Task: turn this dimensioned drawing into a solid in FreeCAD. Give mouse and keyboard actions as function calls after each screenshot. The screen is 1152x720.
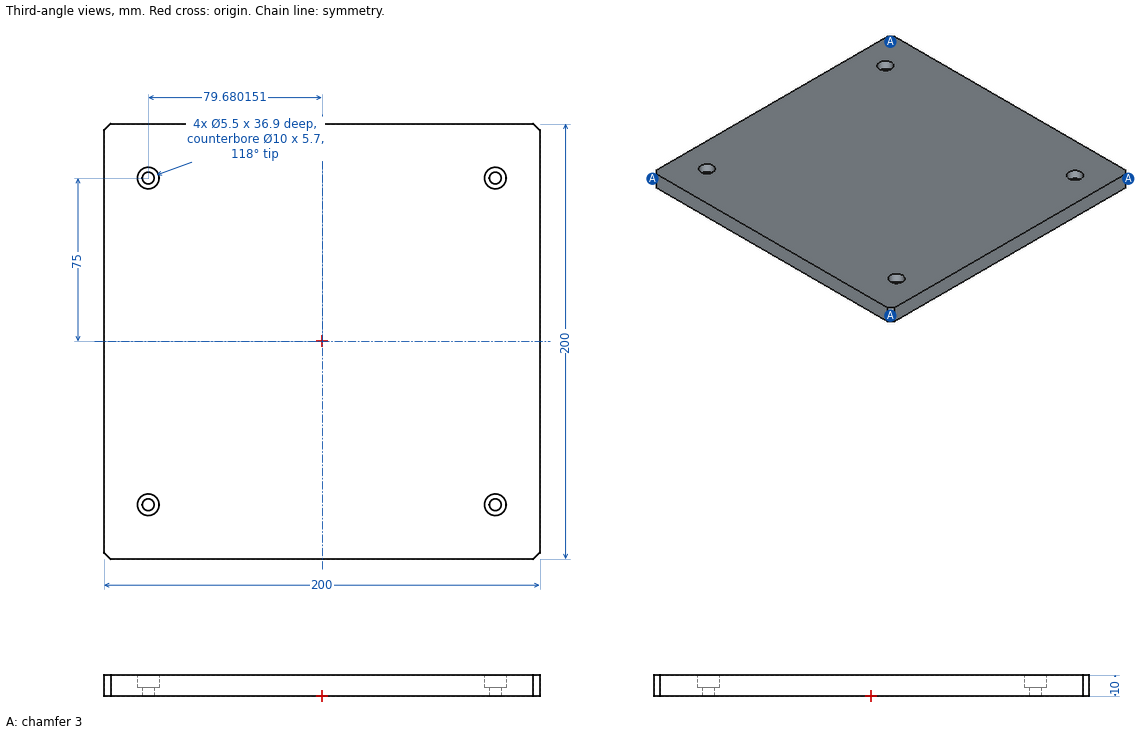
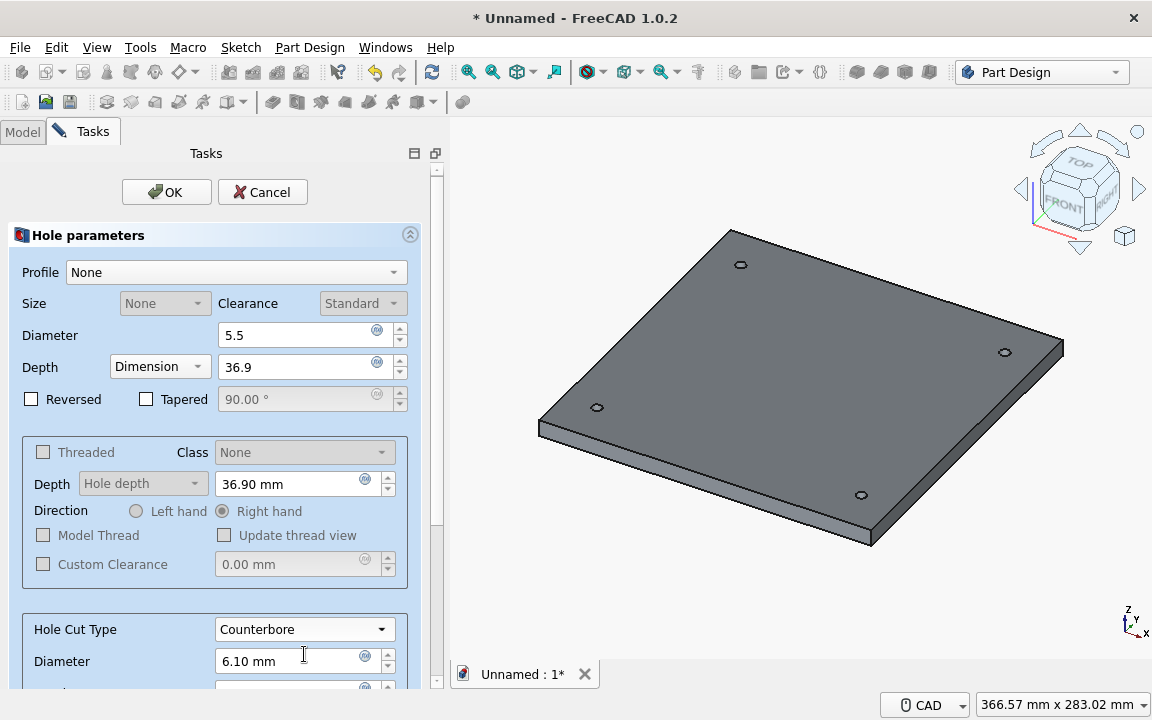
triple_click(298, 661)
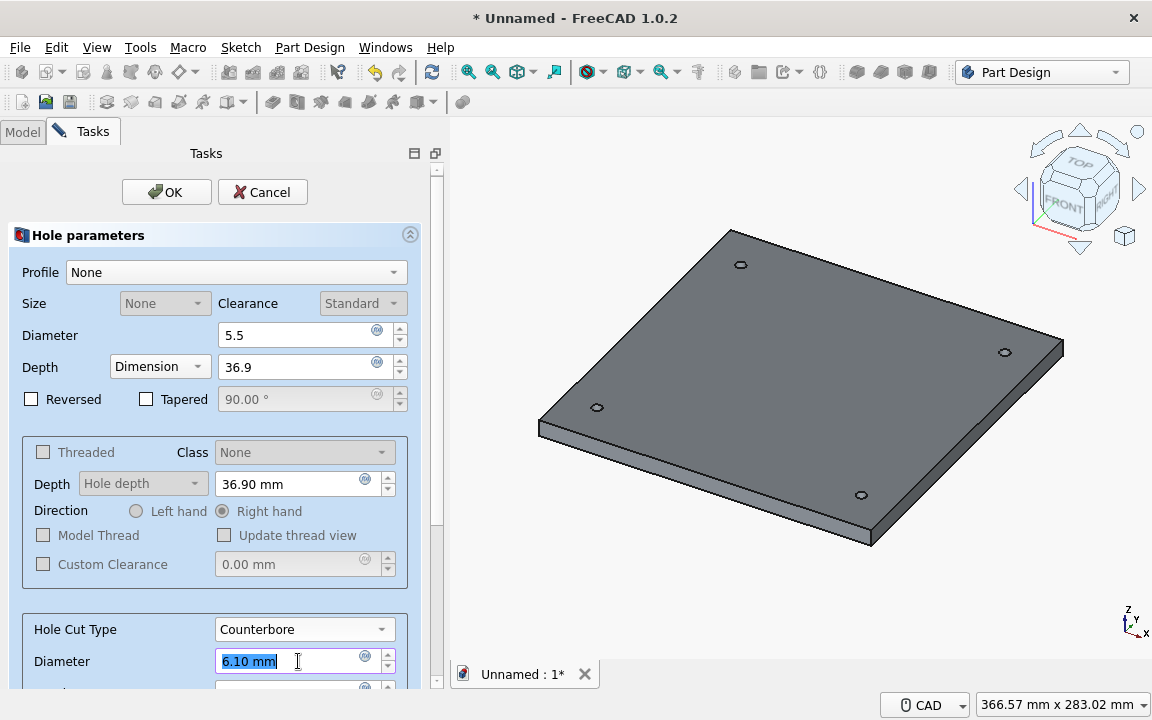
text(10)
key(Tab)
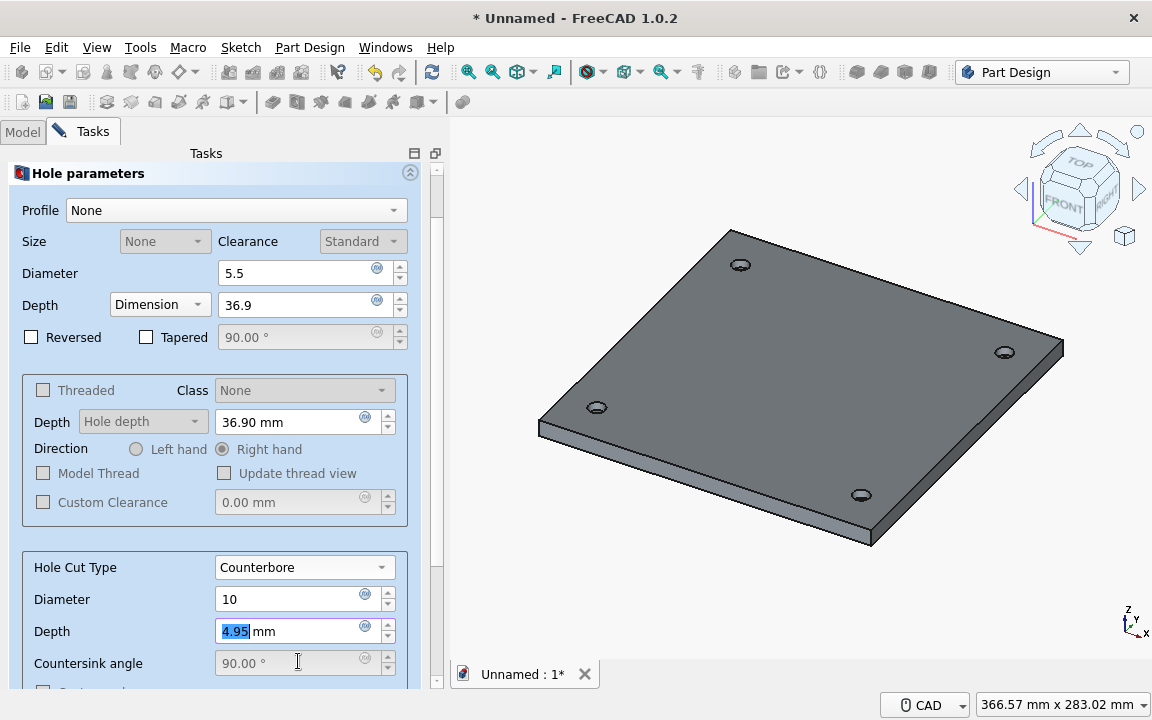
text(5.7)
key(Tab)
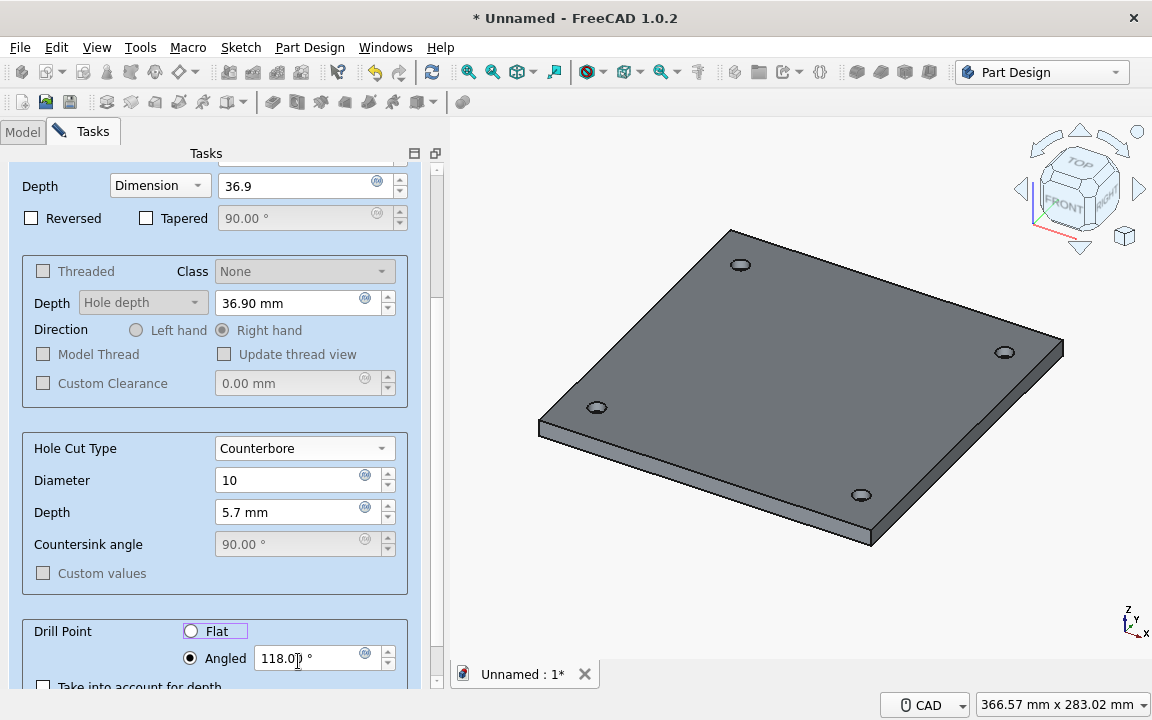
scroll(437, 426, up, 4)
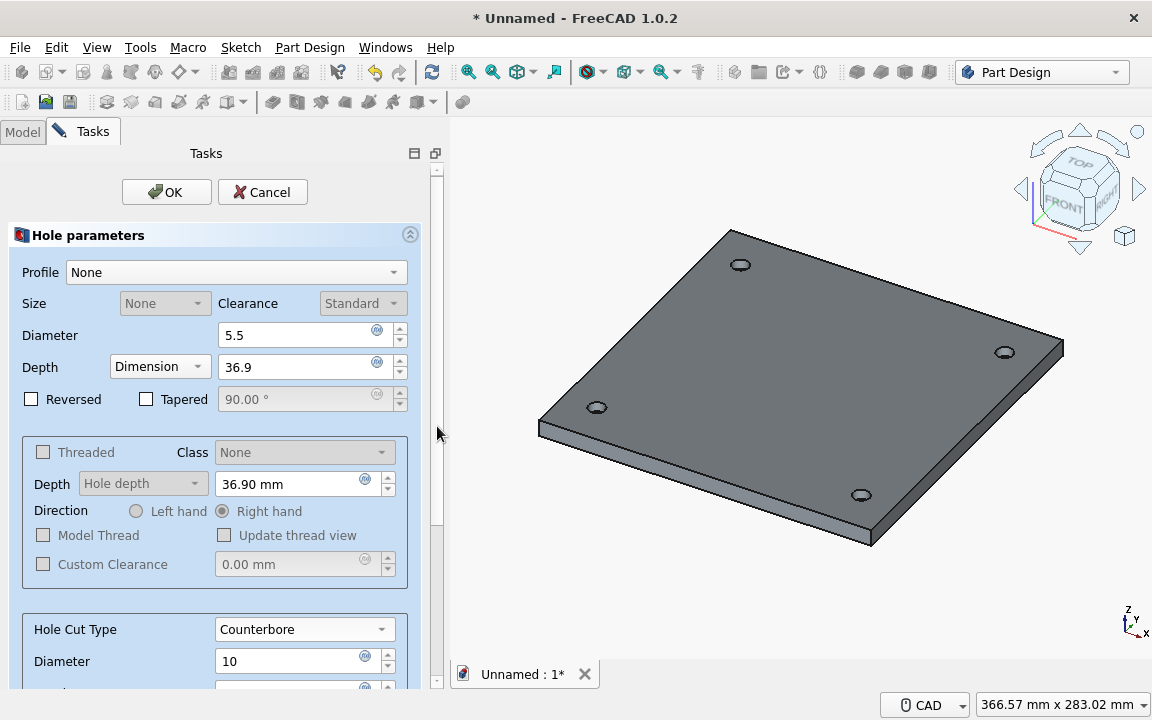
click(167, 192)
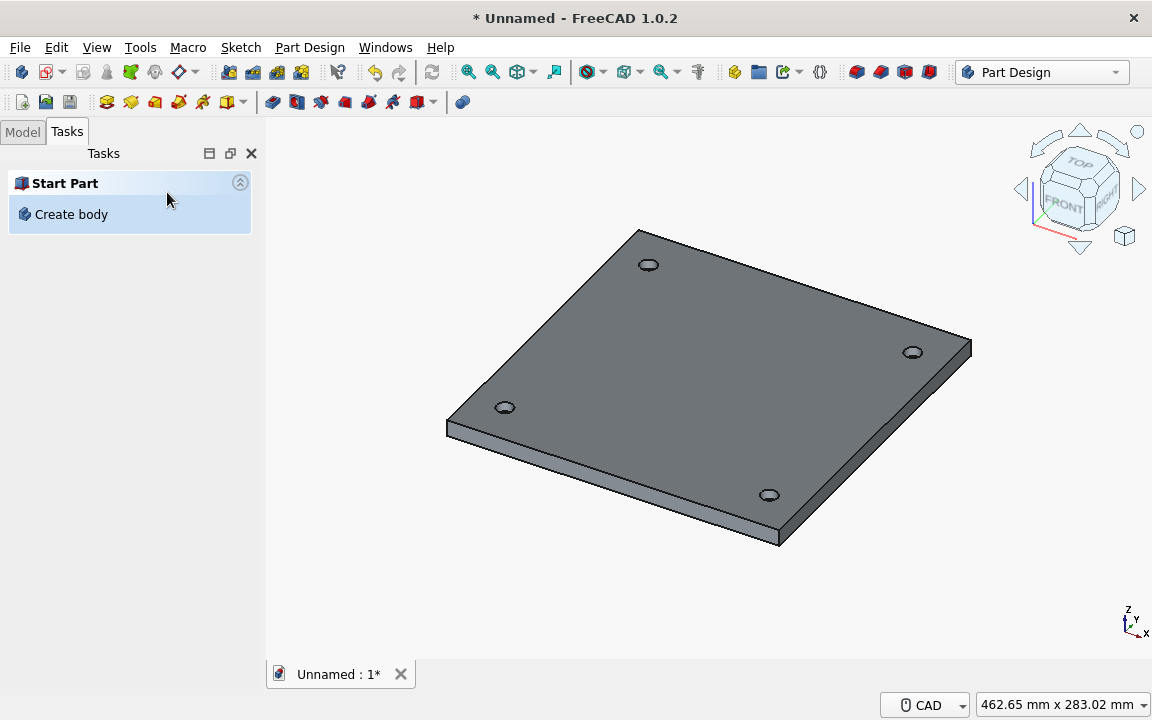
click(779, 537)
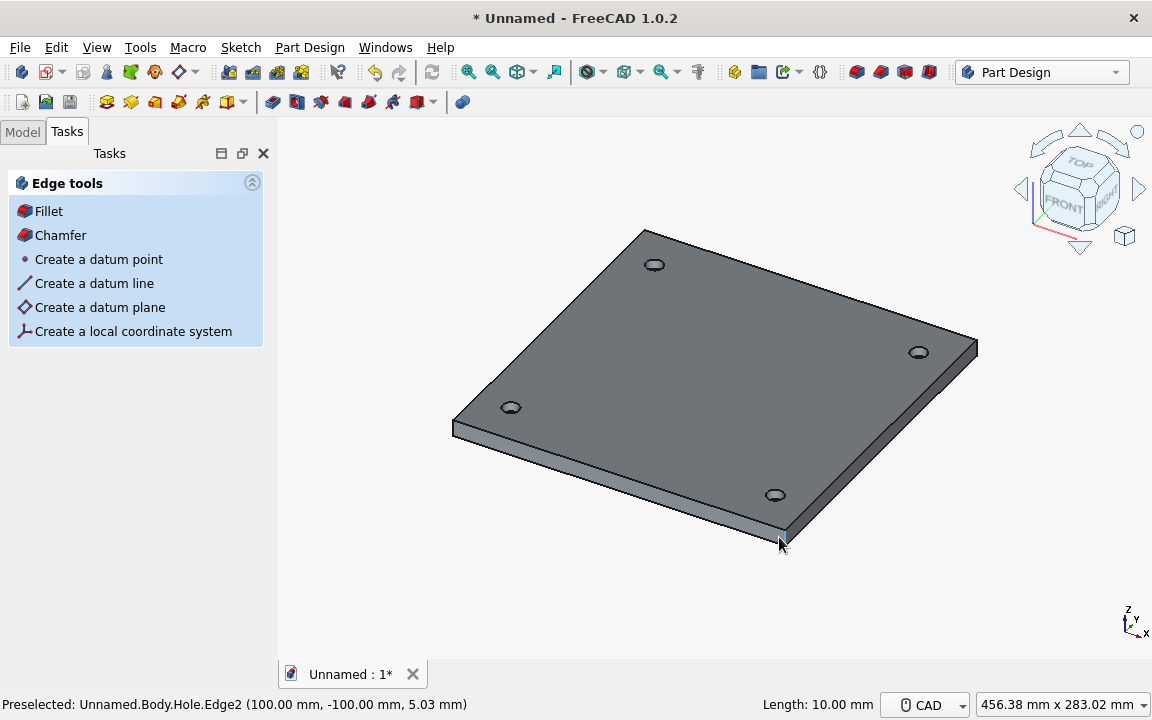
scroll(453, 427, up, 4)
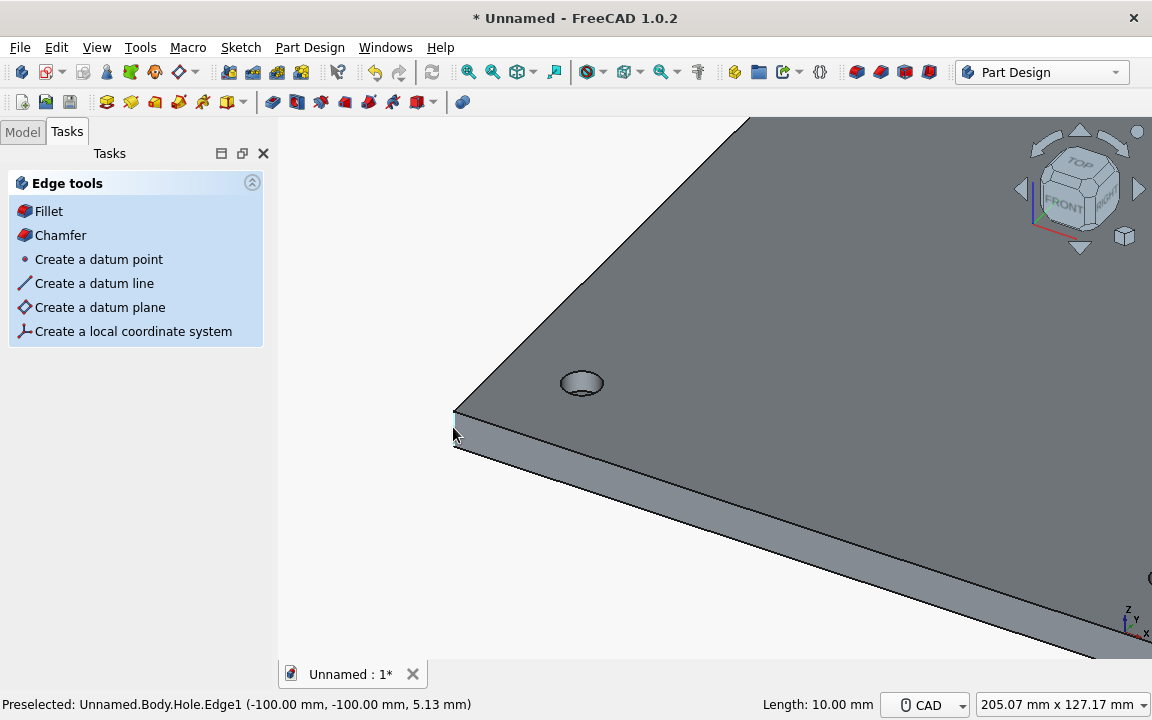
key(v)
key(f)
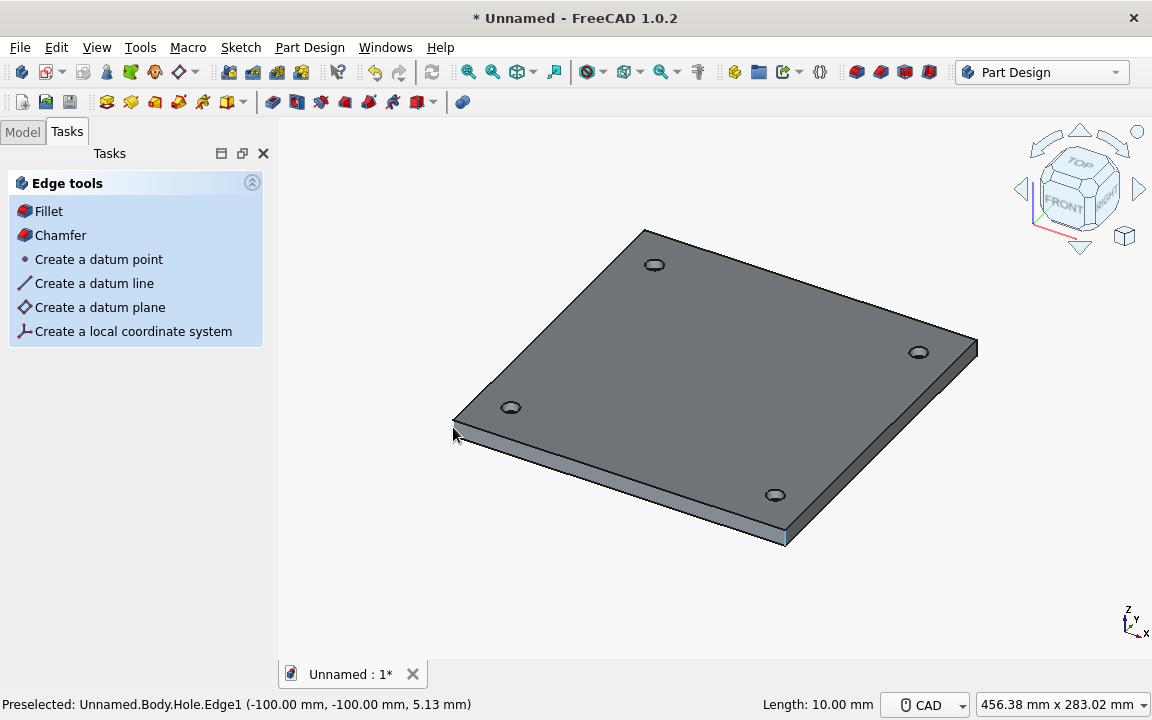
key(0)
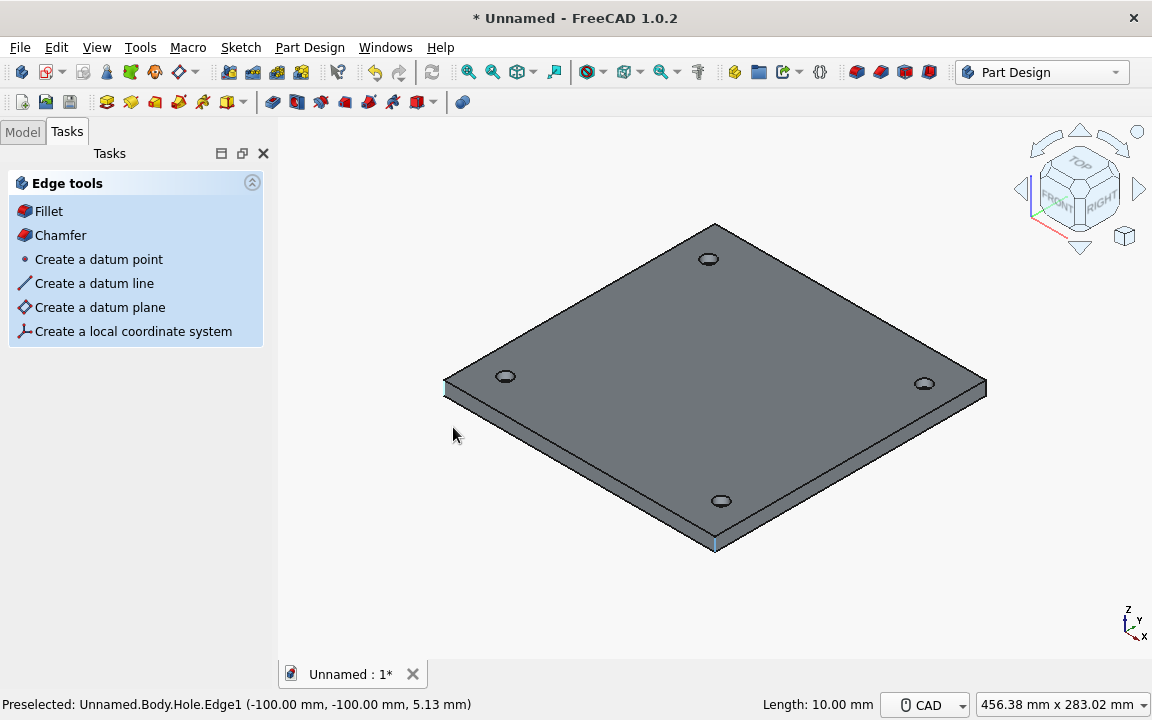
scroll(444, 387, up, 4)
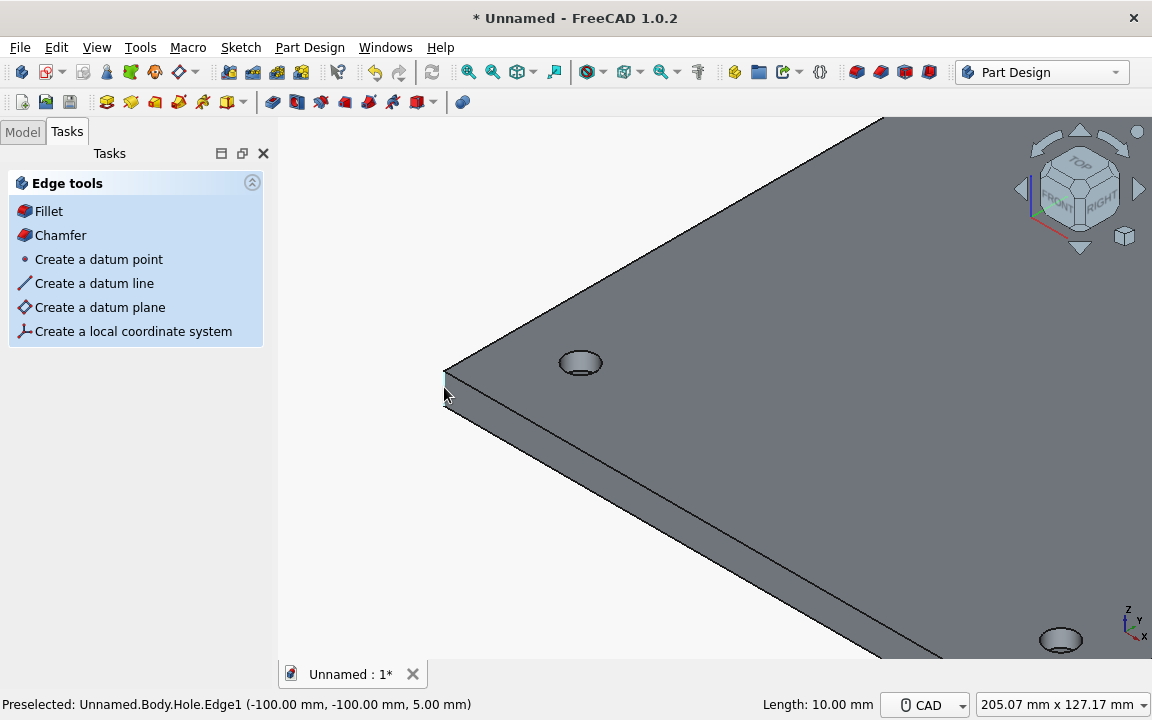
click(470, 72)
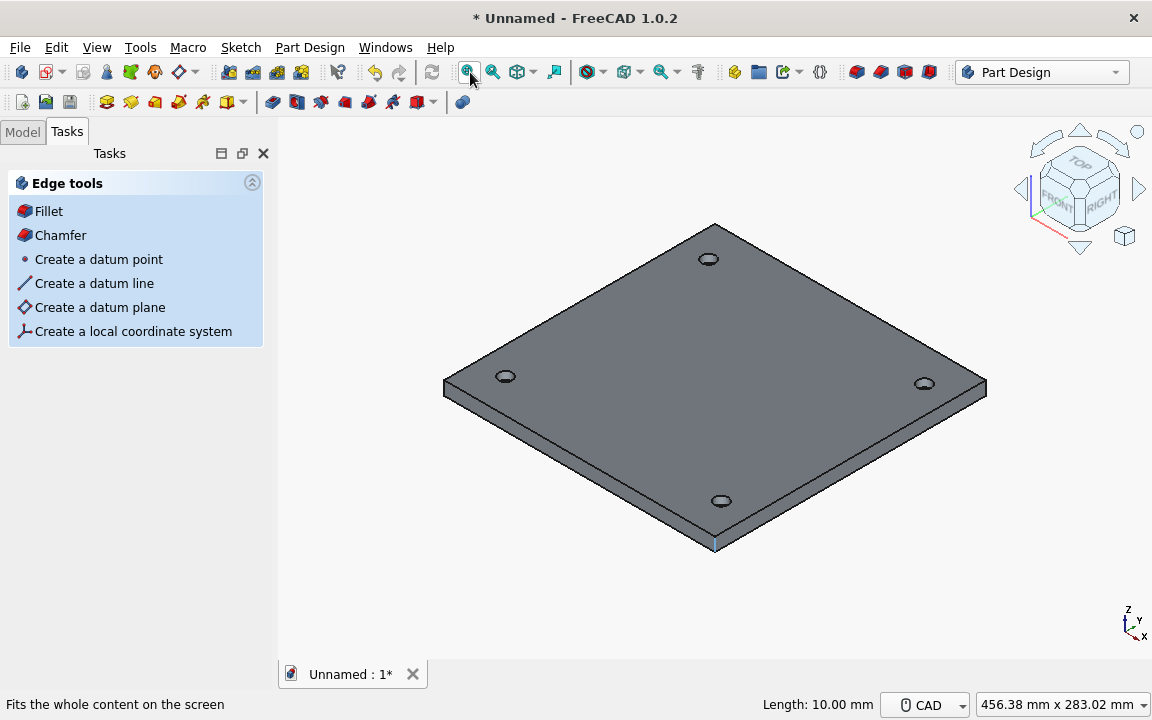
key(2)